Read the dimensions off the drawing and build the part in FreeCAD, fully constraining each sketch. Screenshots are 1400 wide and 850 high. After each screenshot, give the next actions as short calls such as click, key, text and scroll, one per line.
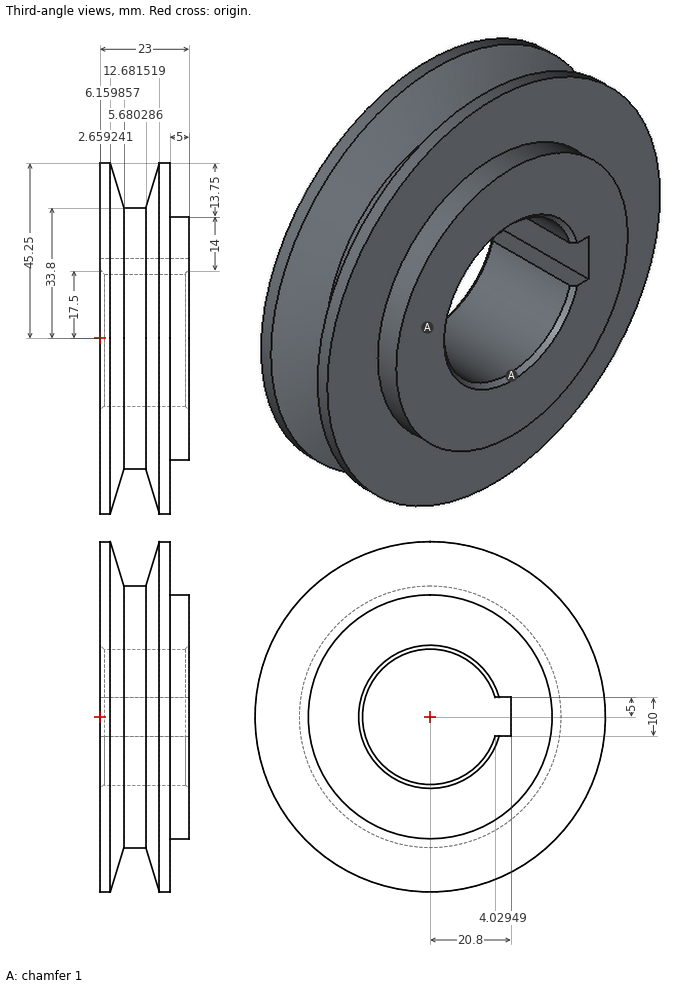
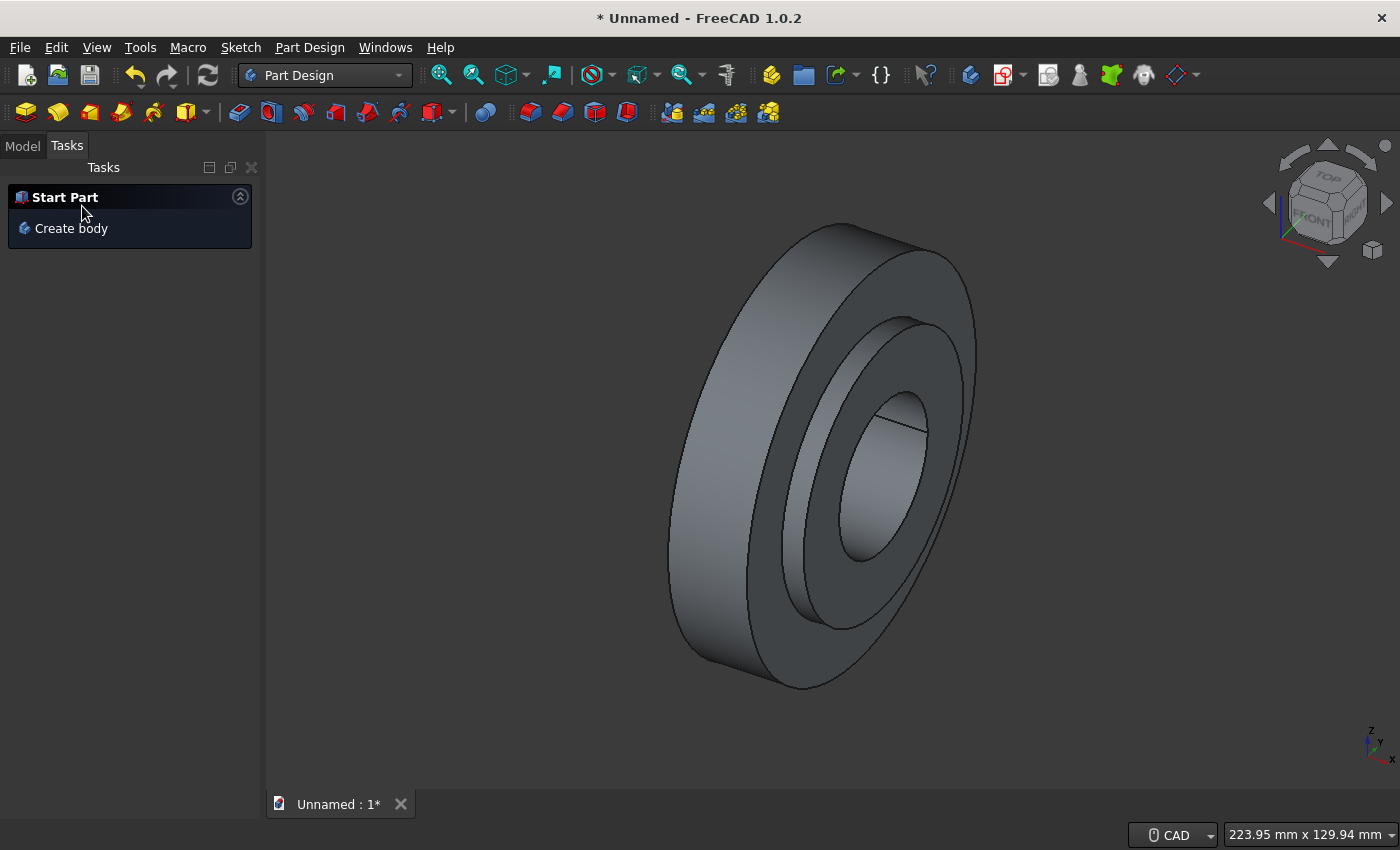
click(1004, 76)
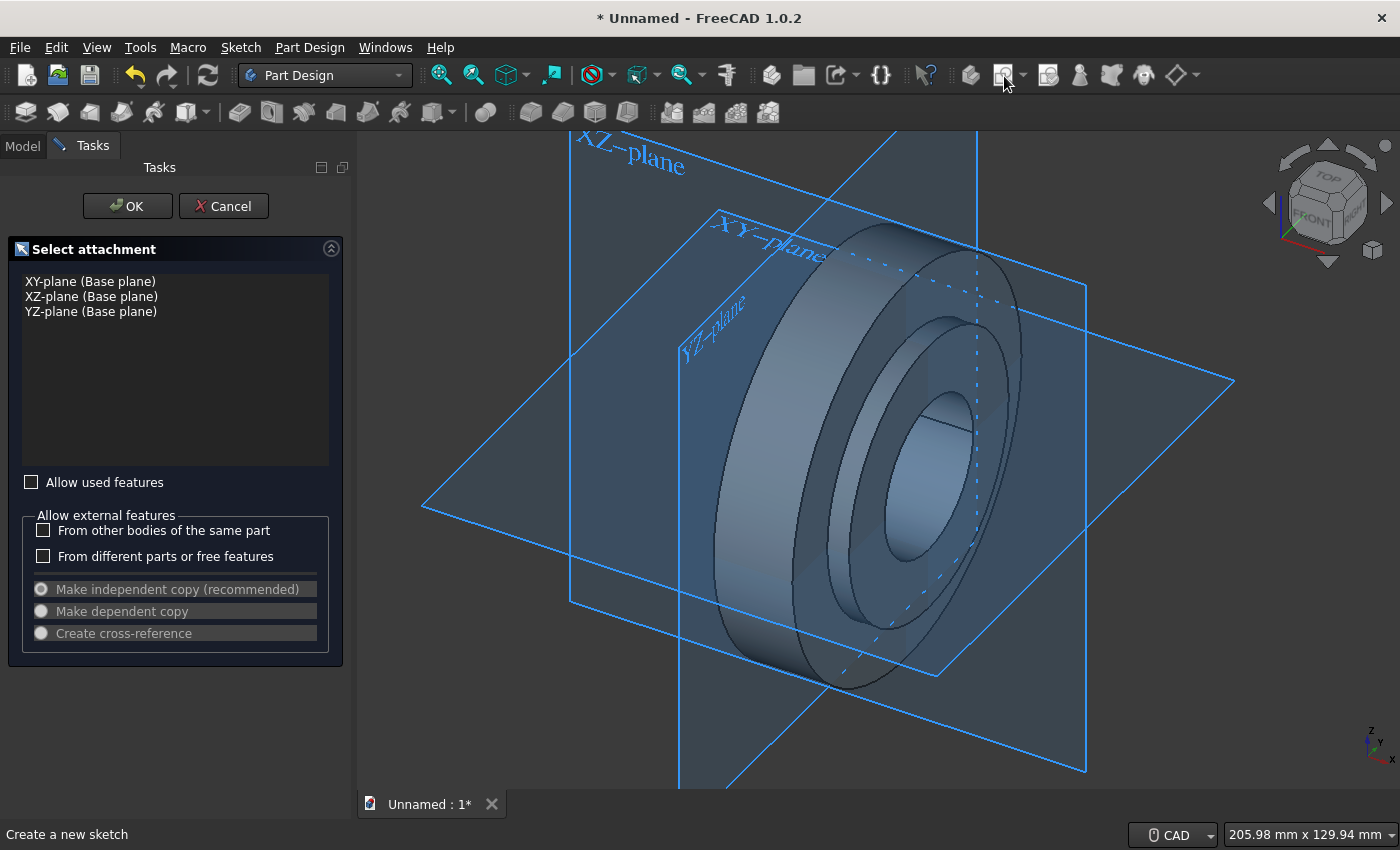
click(82, 282)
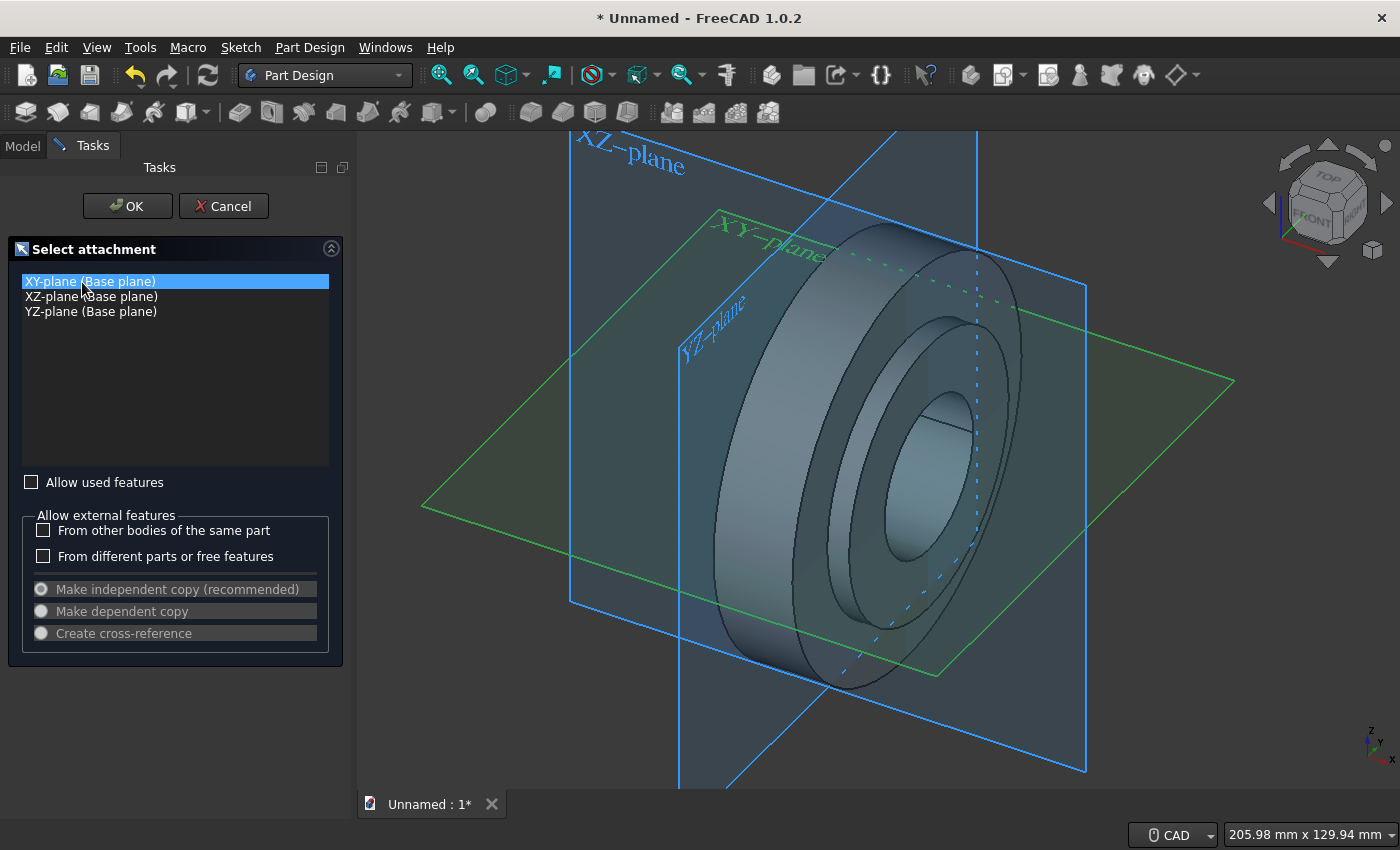
click(128, 206)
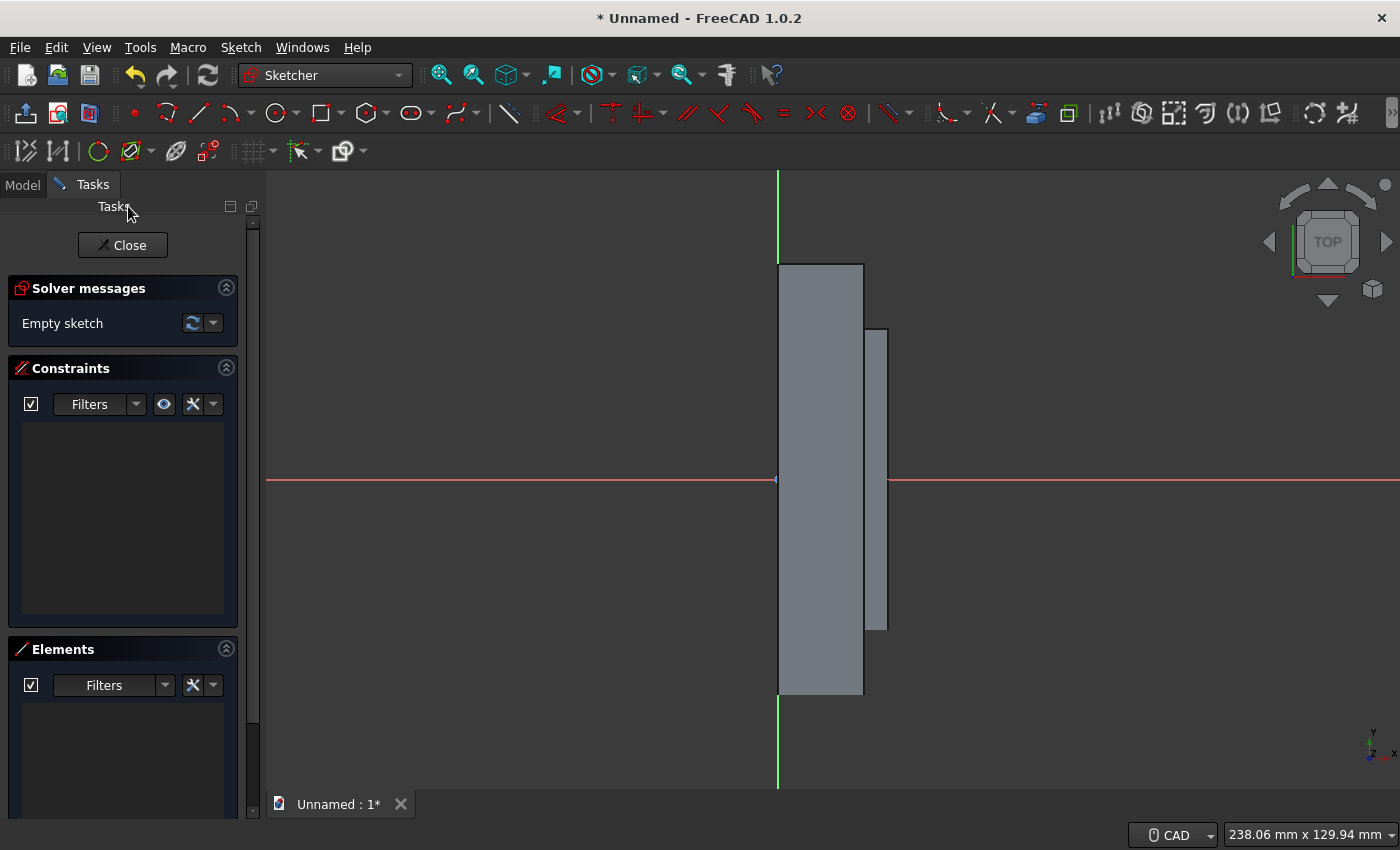
key(q)
key(s)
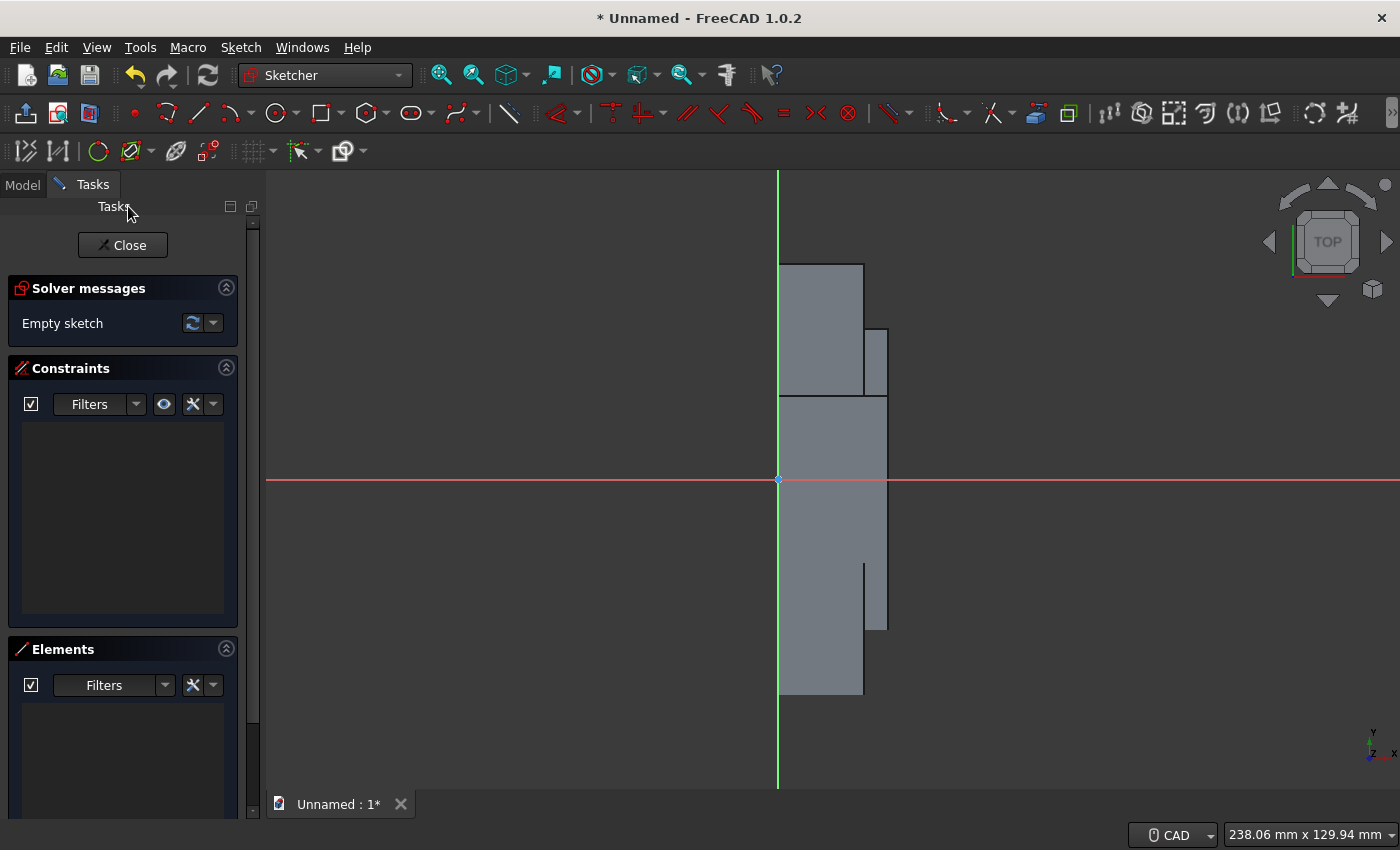
scroll(830, 262, up, 10)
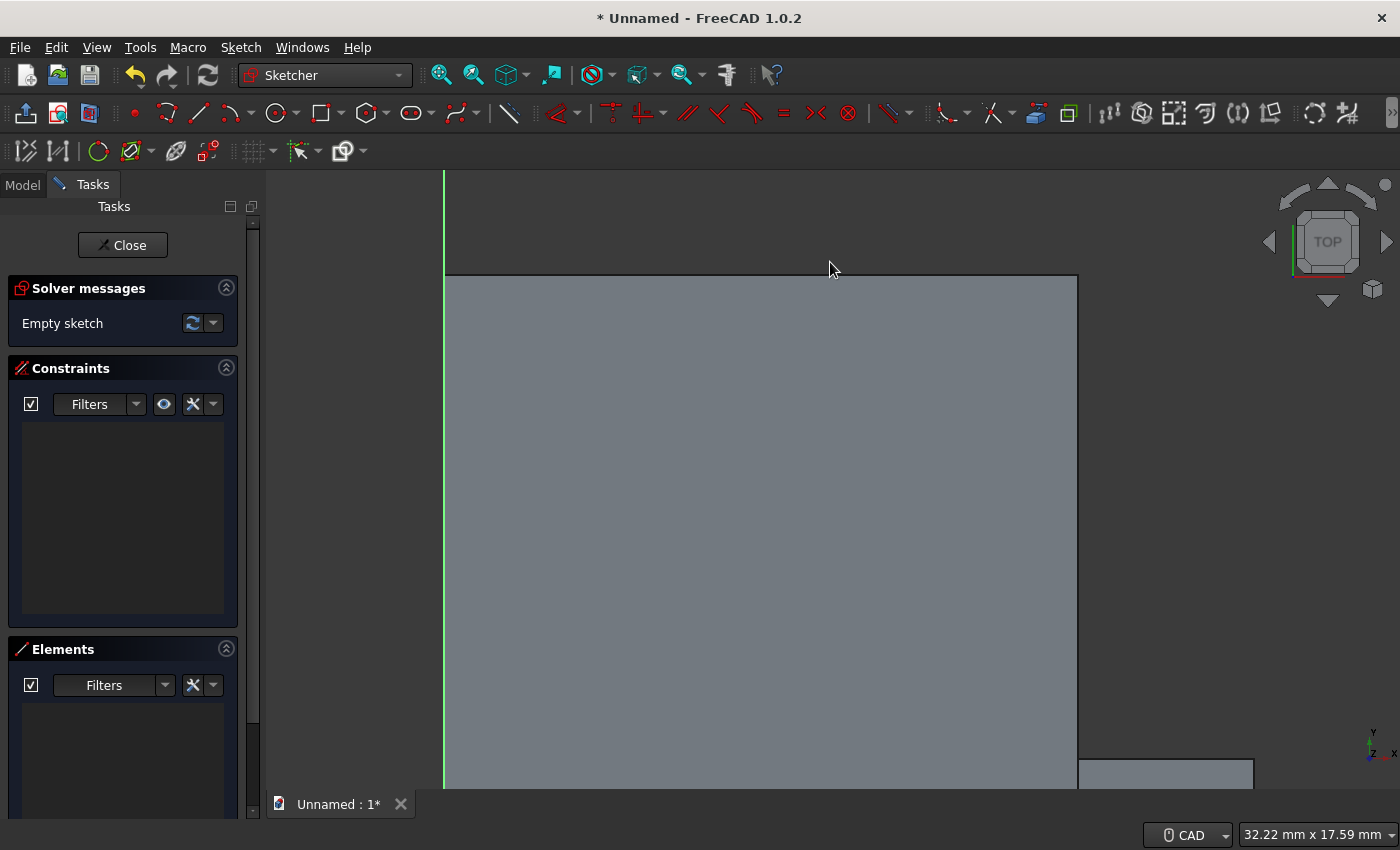
key(g)
key(m)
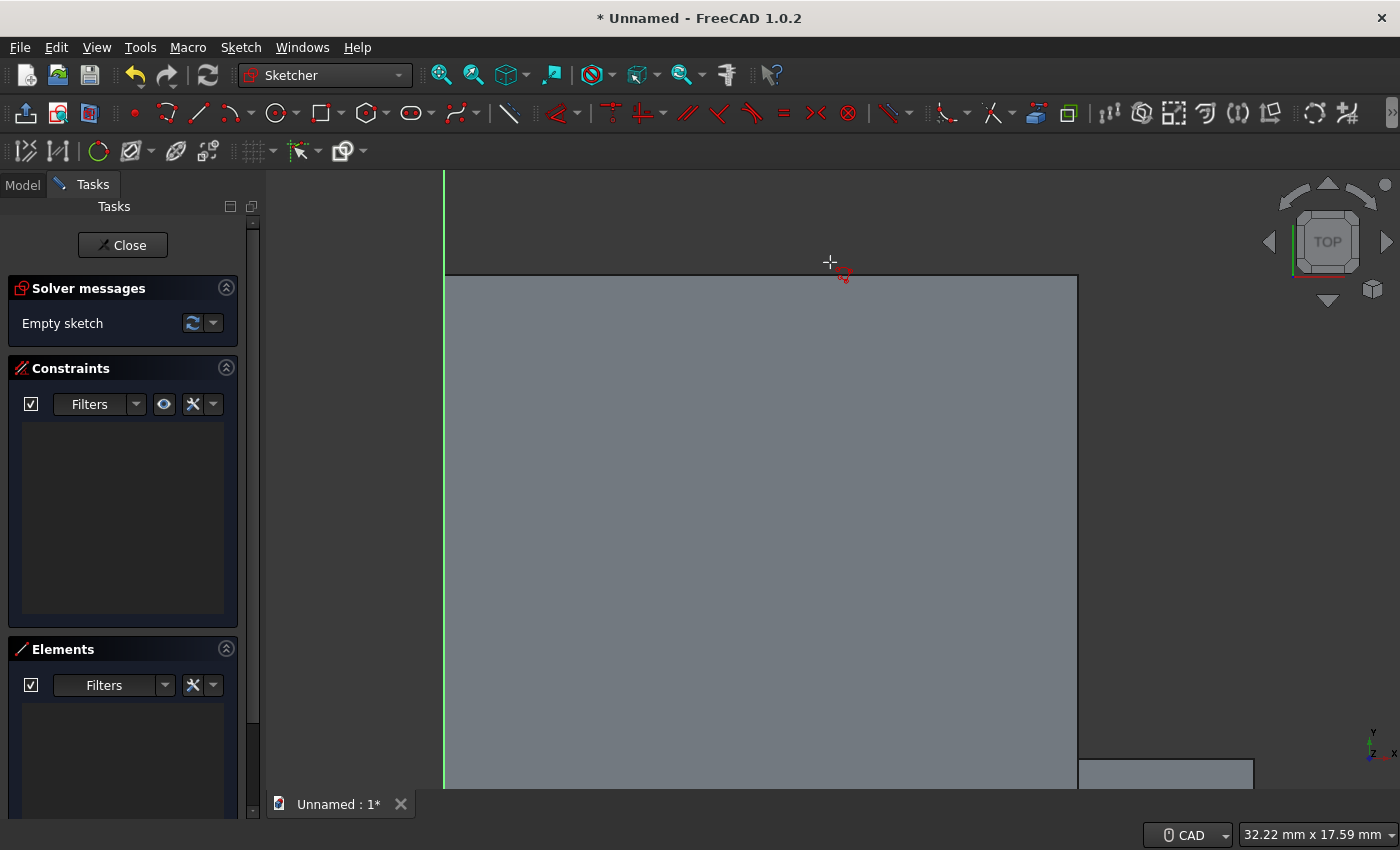
click(661, 678)
click(861, 678)
click(984, 275)
click(538, 275)
click(661, 679)
key(Escape)
key(Escape)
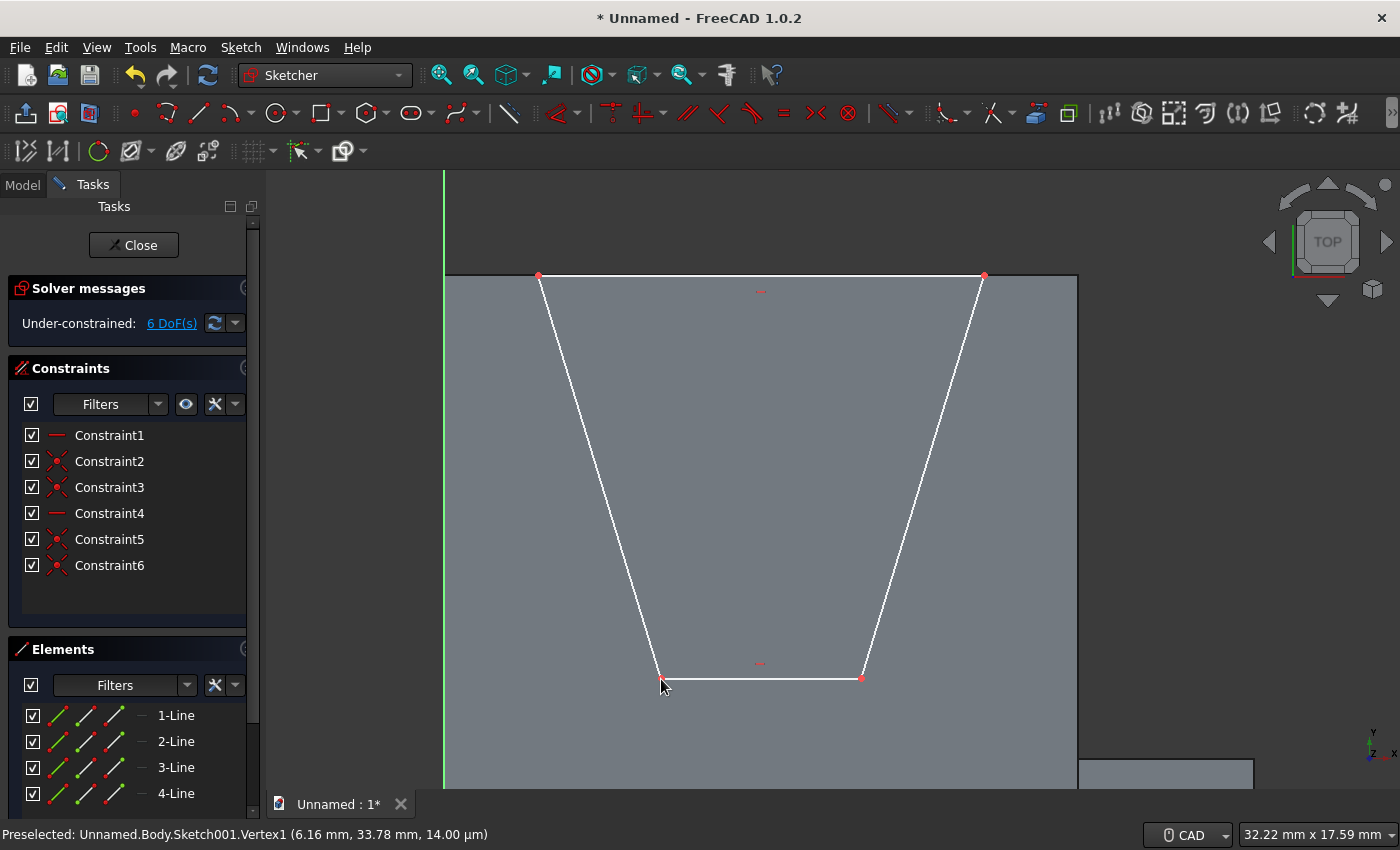
key(d)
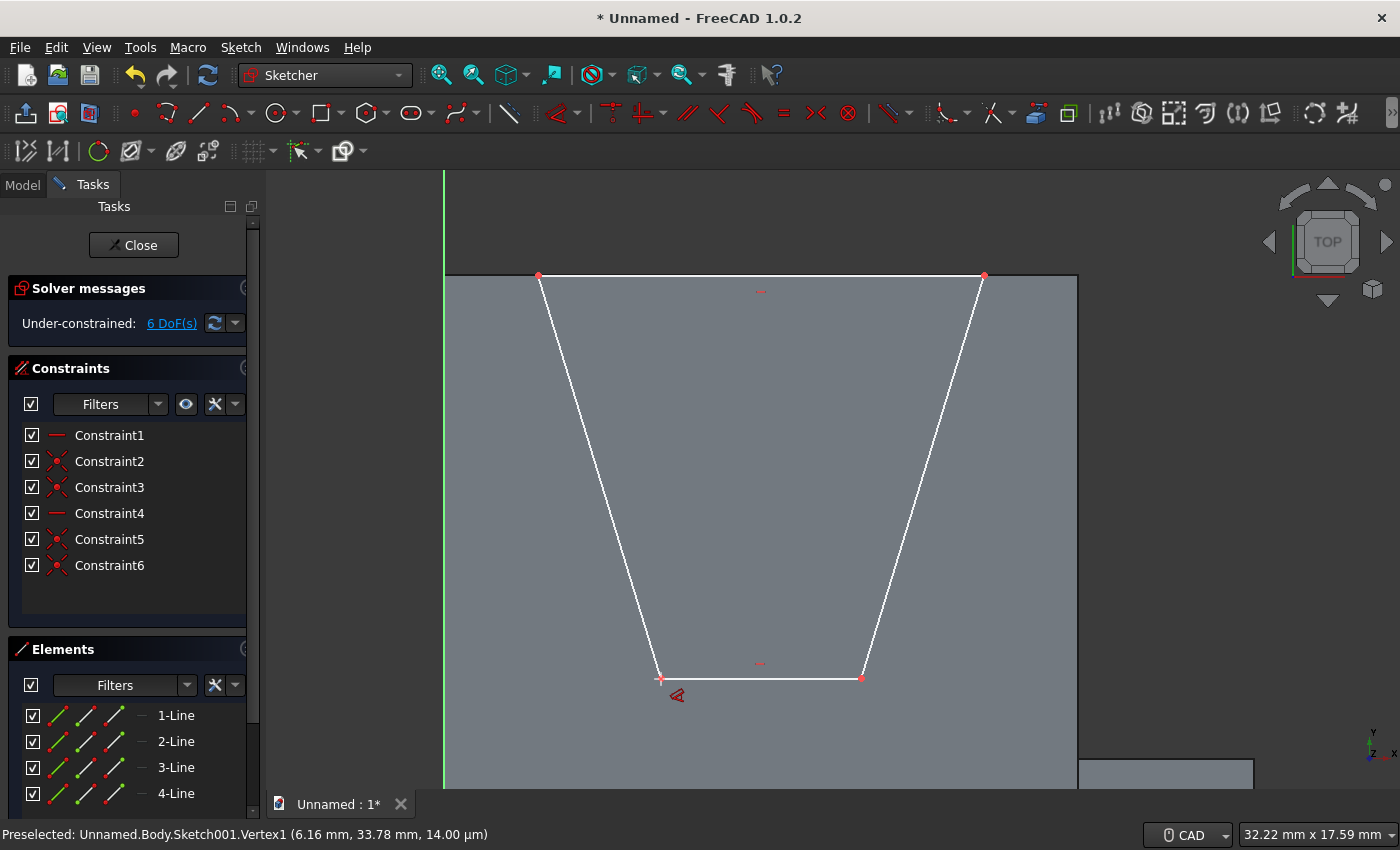
click(661, 679)
click(410, 720)